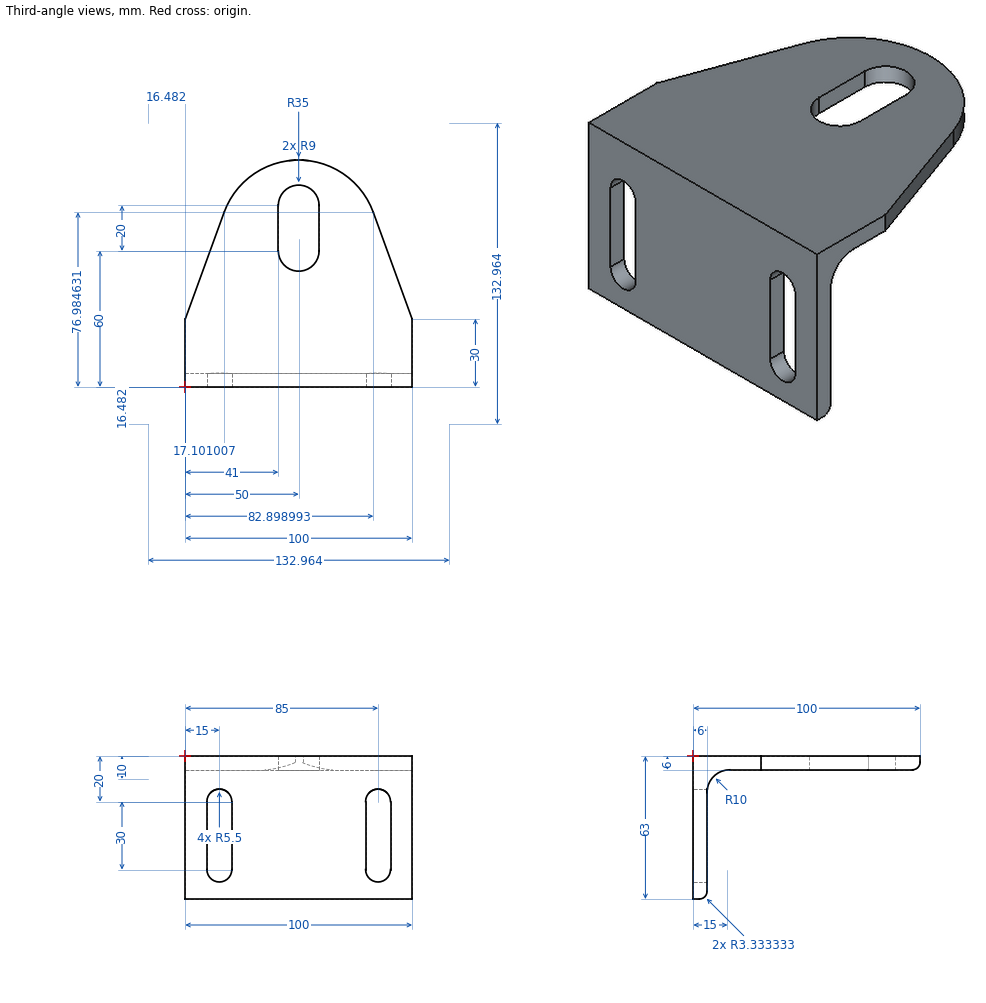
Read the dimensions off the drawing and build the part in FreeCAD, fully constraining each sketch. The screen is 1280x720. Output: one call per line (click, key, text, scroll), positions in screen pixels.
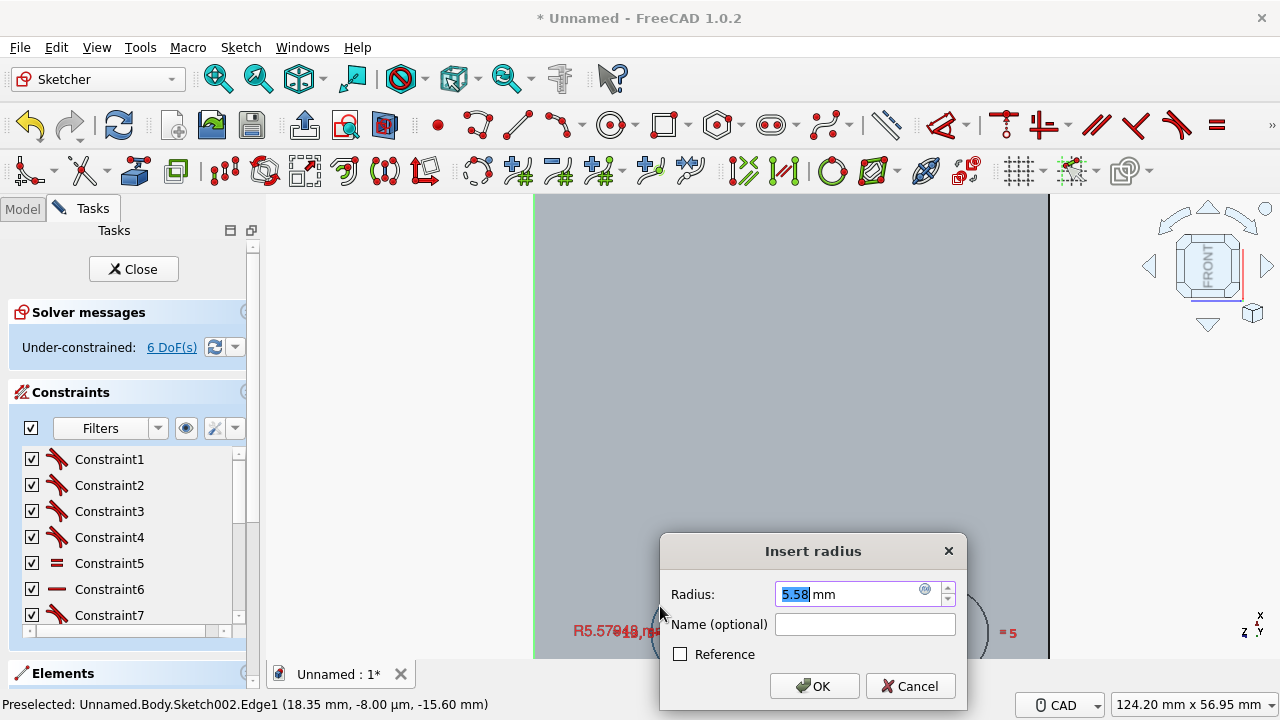
text(5.5)
key(Return)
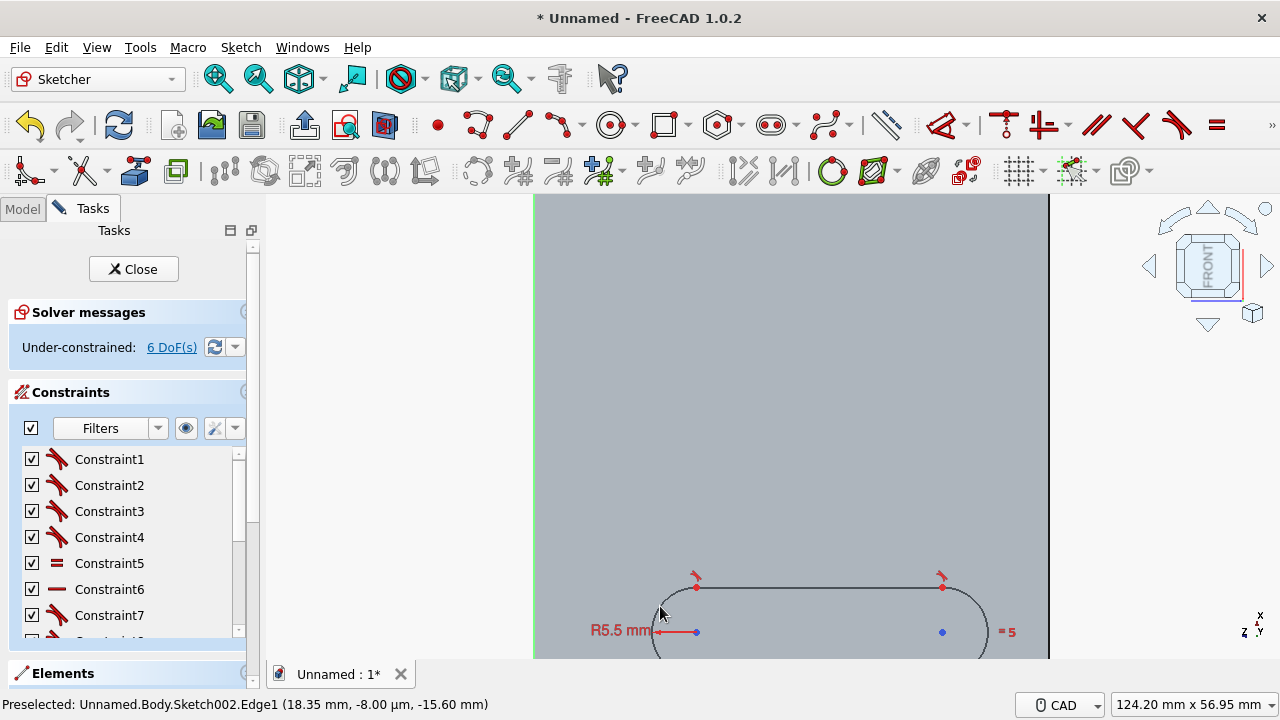
click(771, 588)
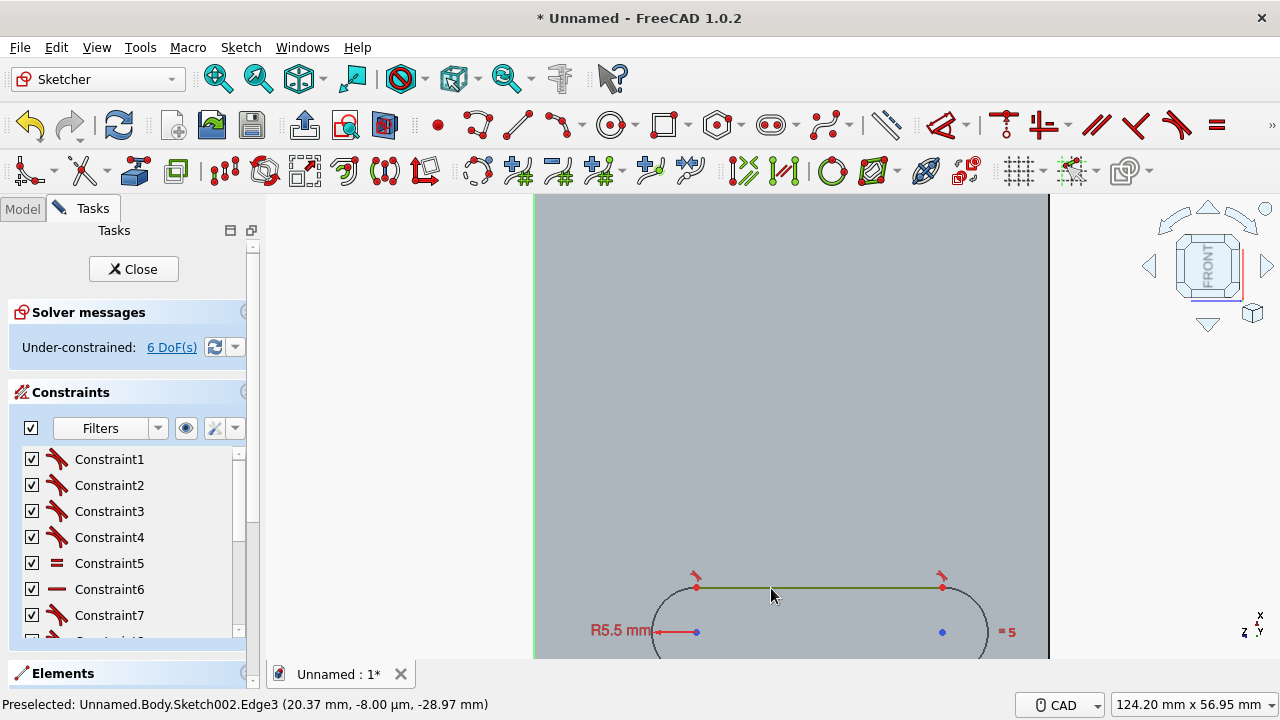
key(l)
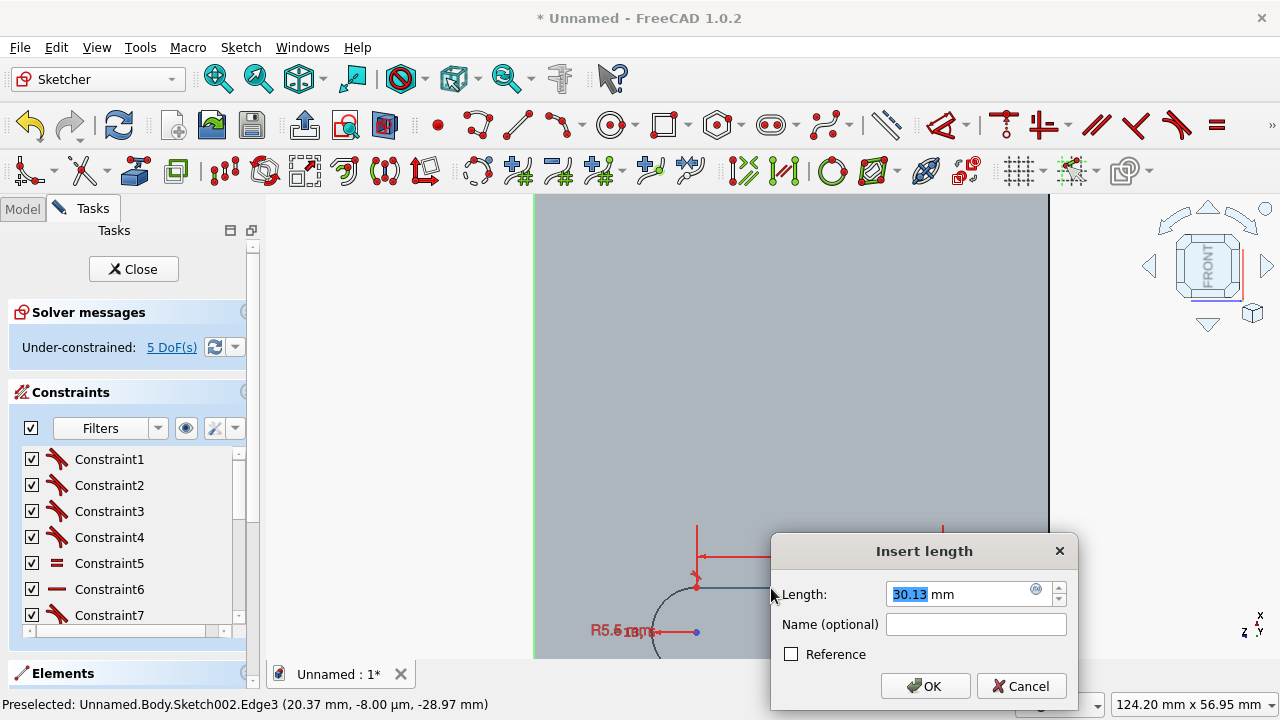
text(30)
key(Return)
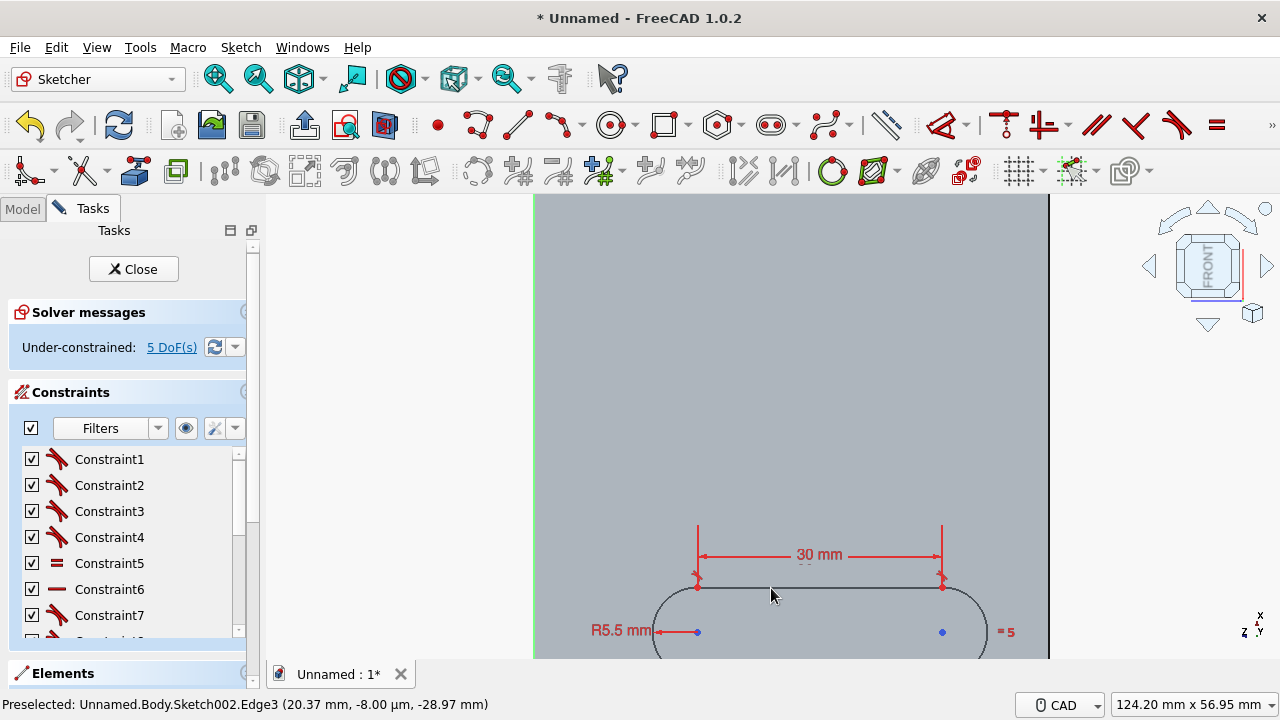
scroll(672, 451, down, 5)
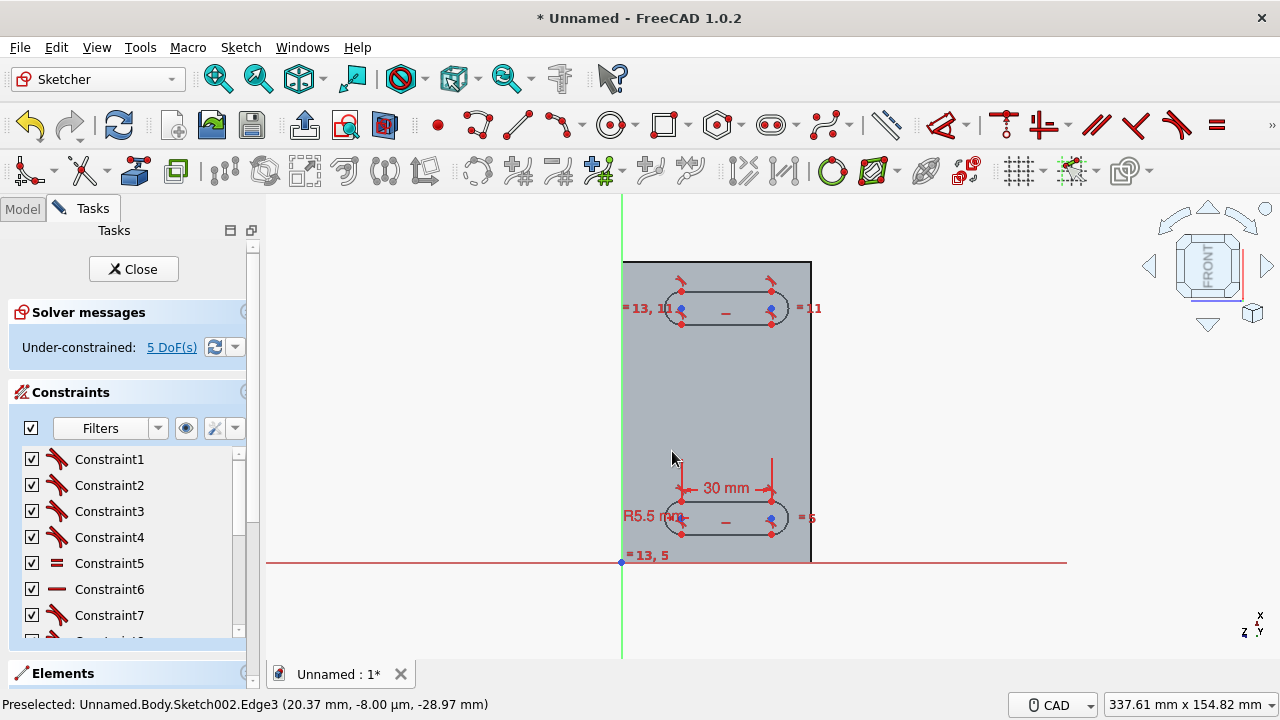
click(709, 292)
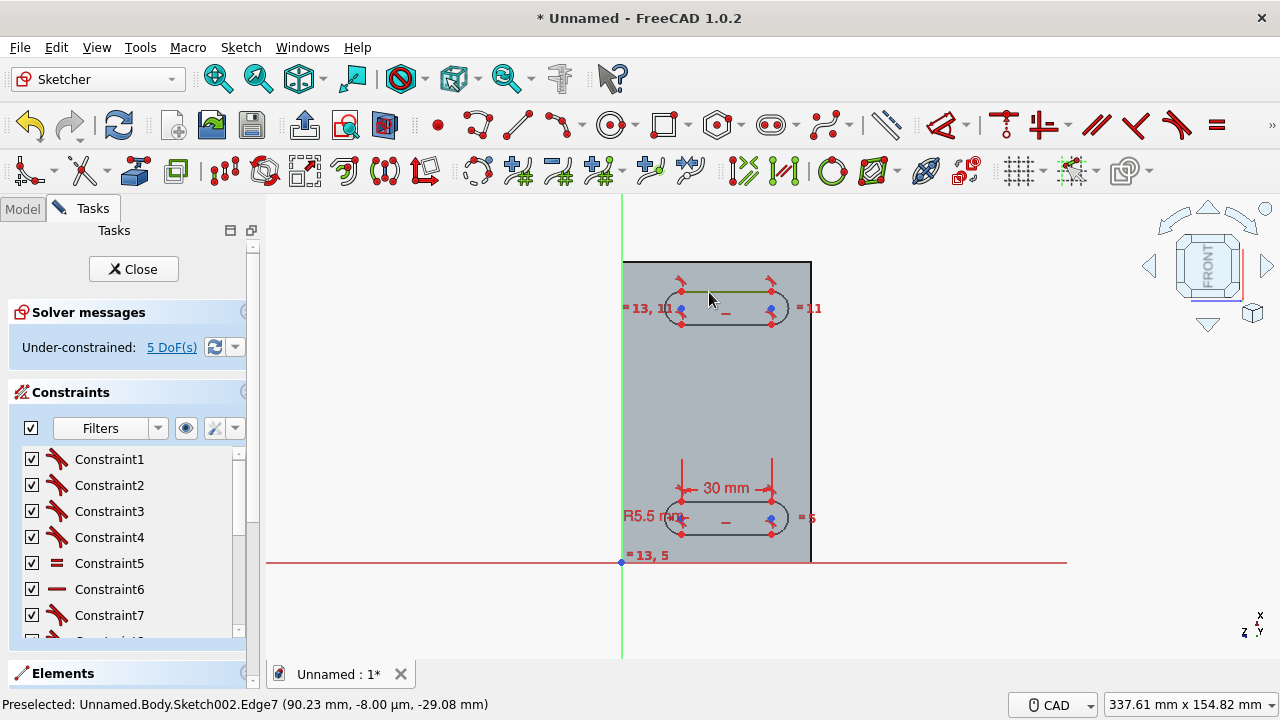
key(l)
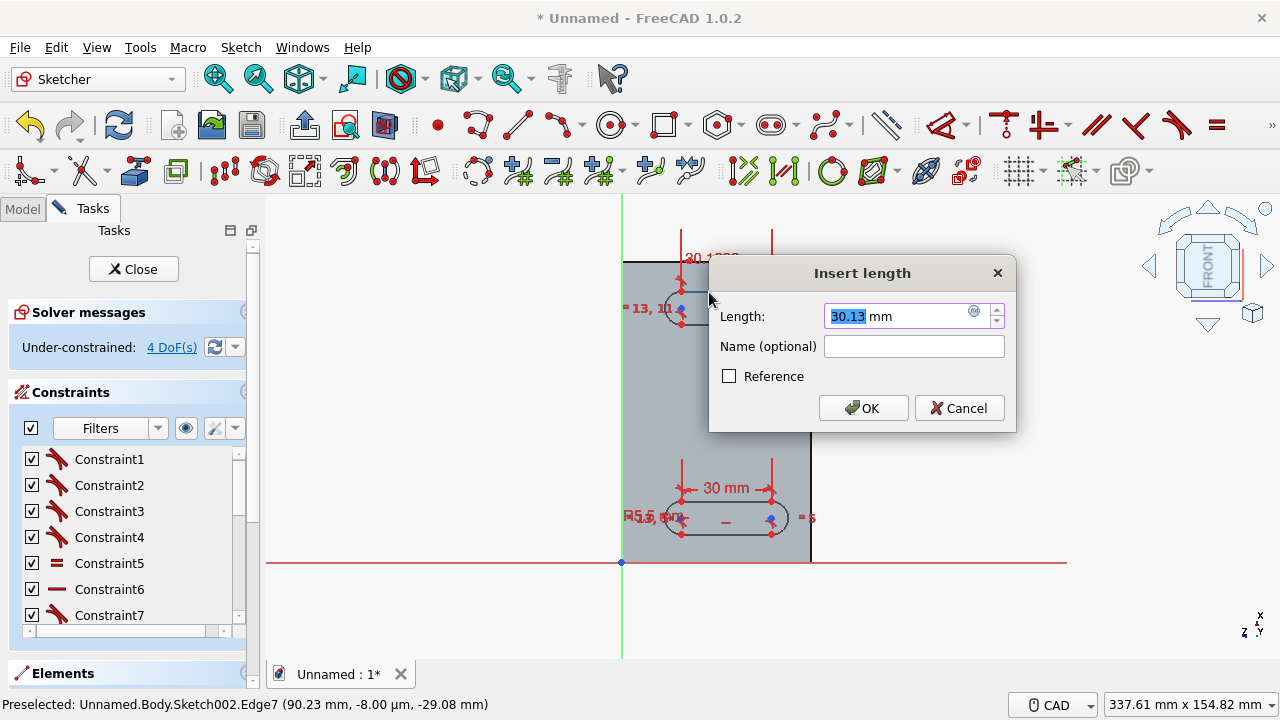
text(30)
key(Return)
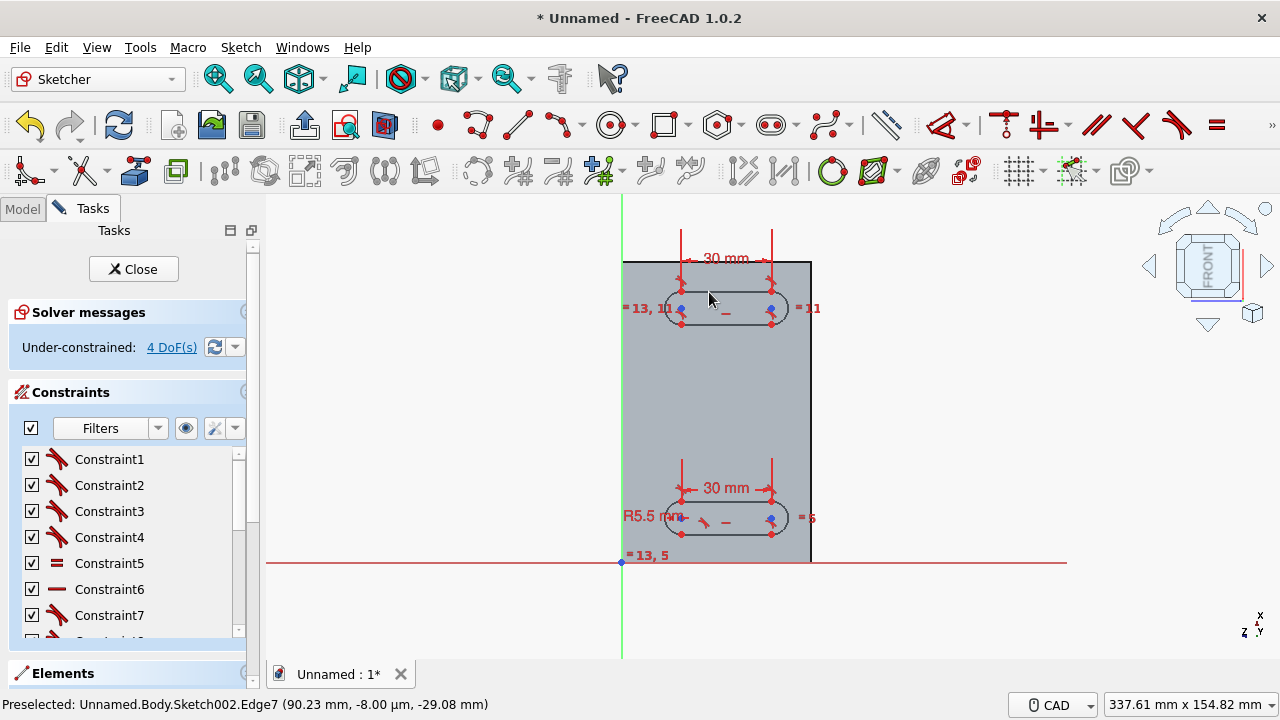
click(682, 502)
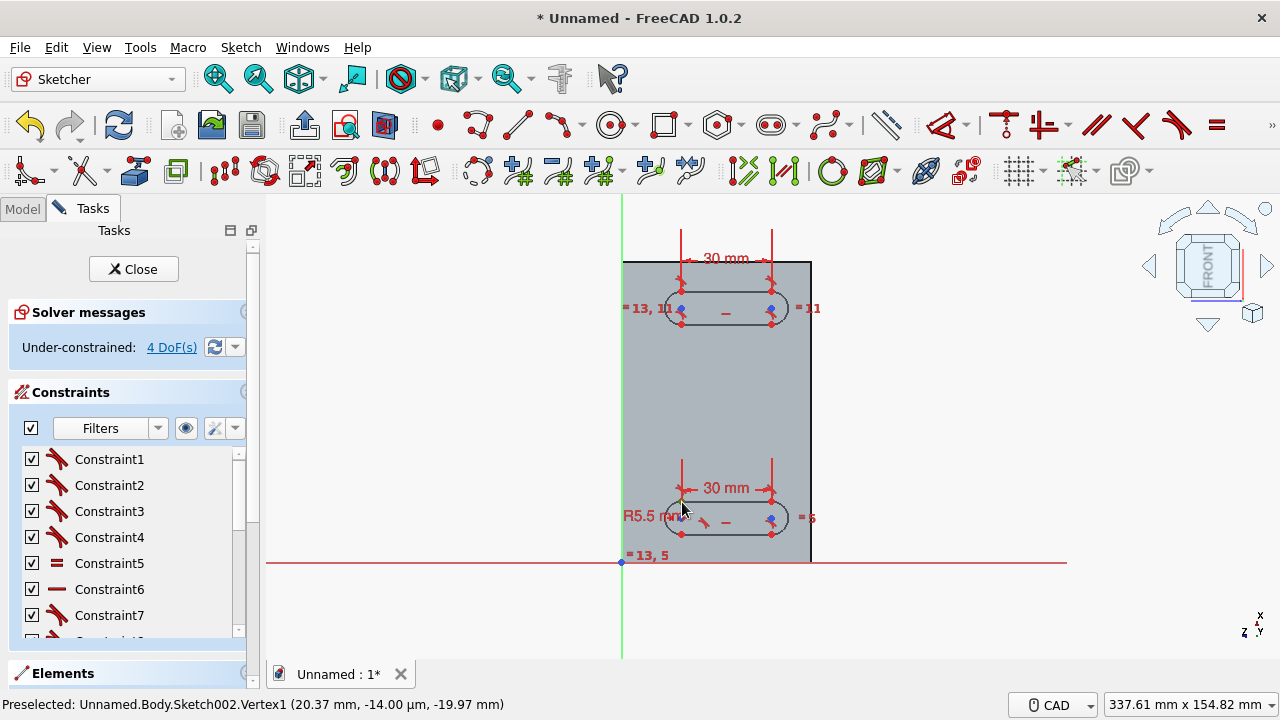
key(l)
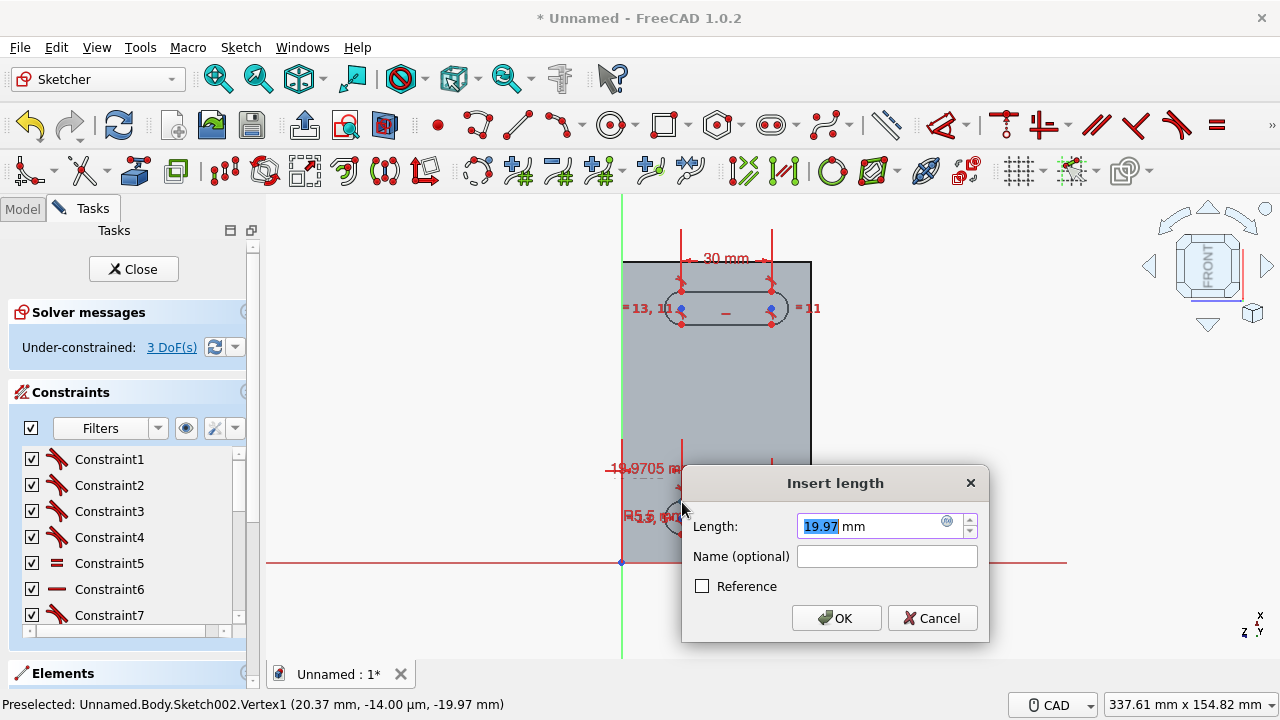
text(20)
key(Return)